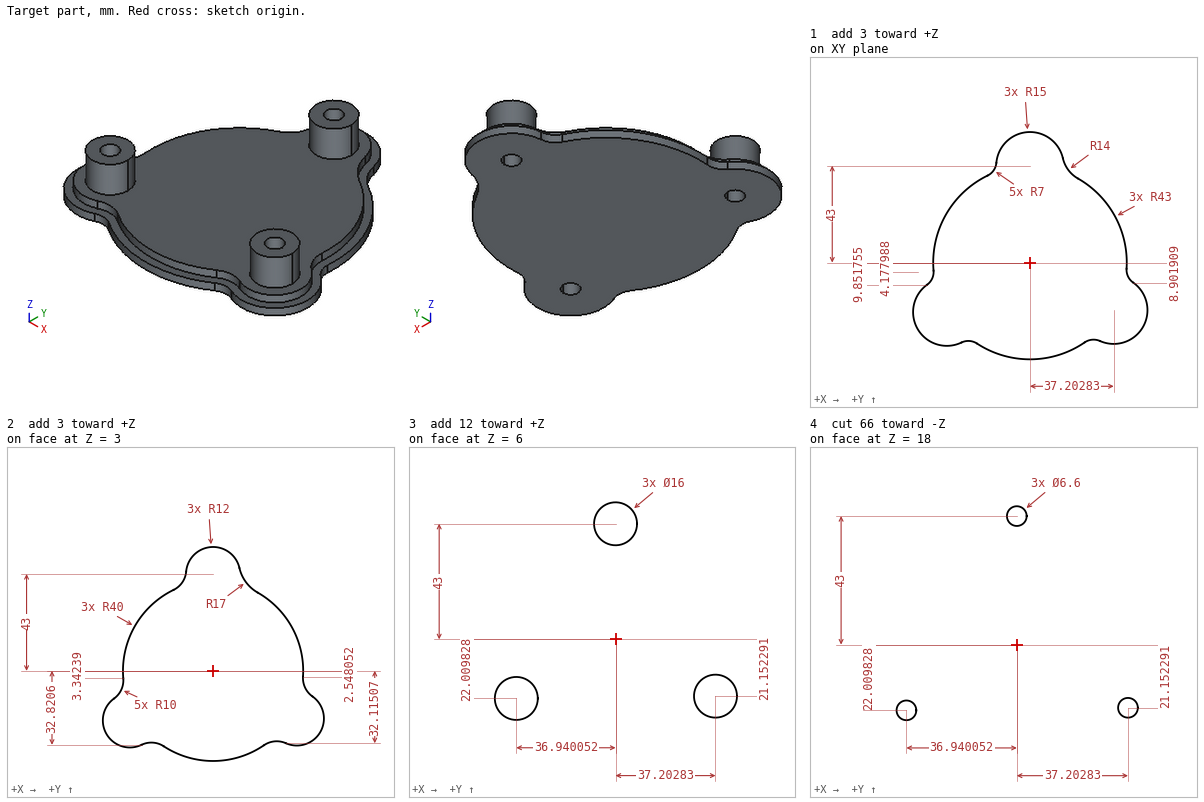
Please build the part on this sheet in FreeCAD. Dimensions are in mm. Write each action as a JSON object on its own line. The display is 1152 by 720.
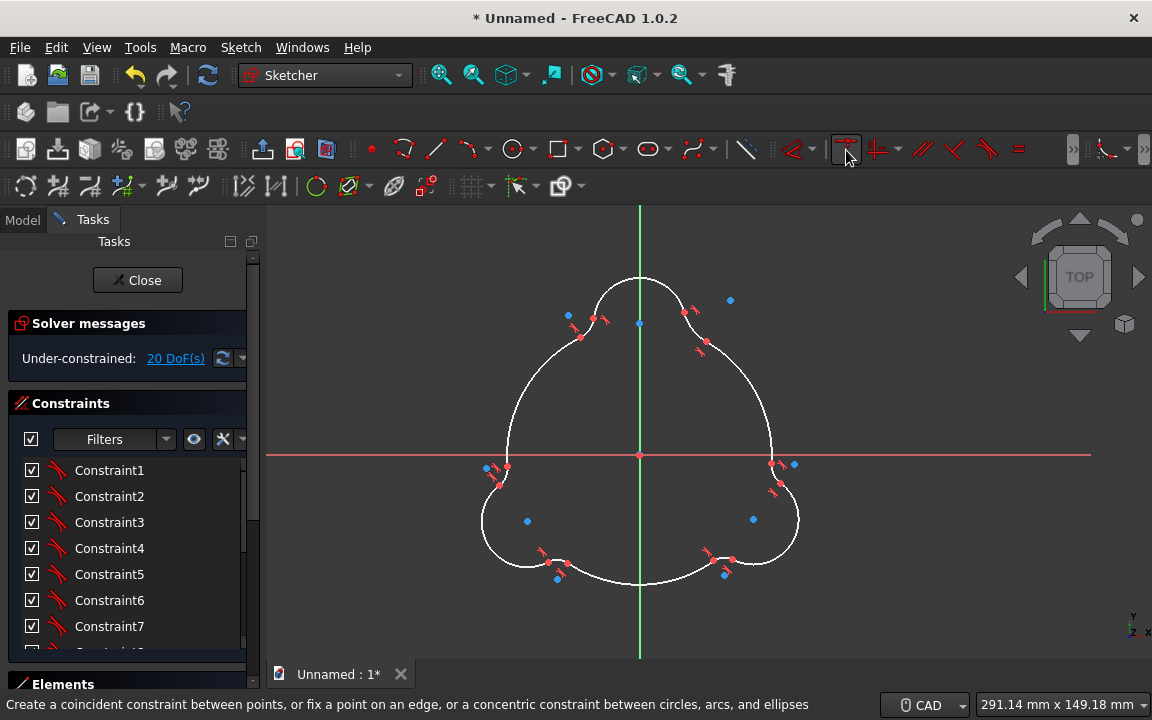
{"action": "scroll", "coordinate": [640, 455], "scroll_direction": "up", "scroll_amount": 4}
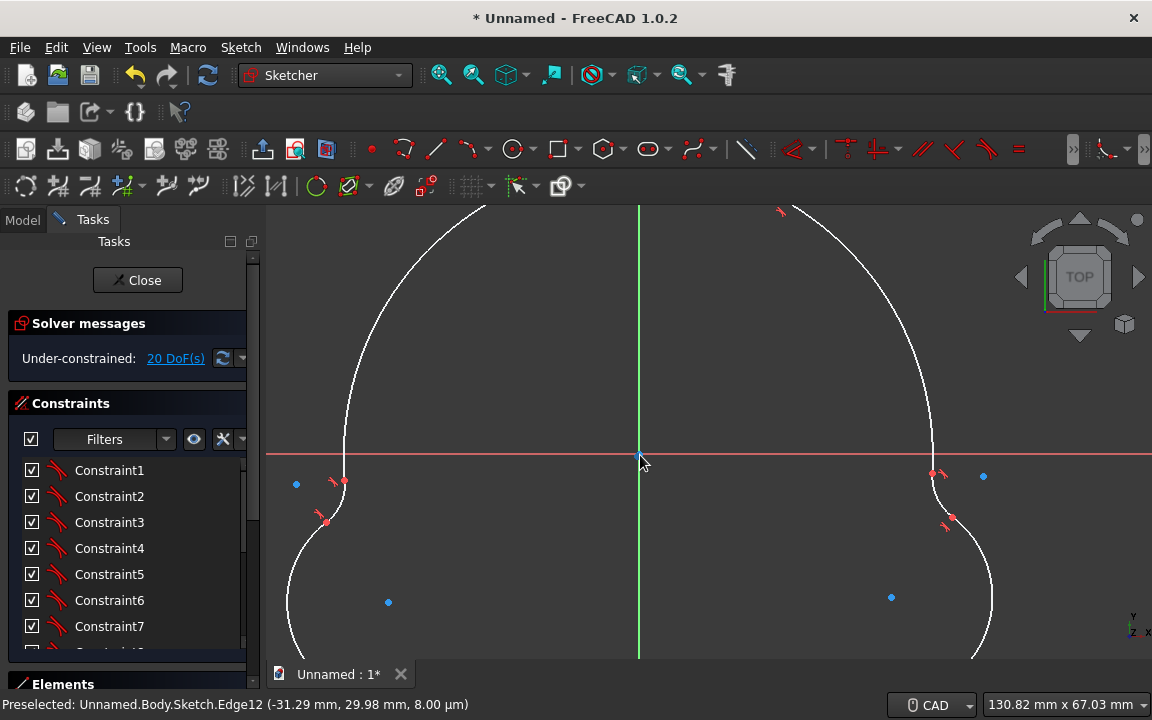
{"action": "left_click_drag", "start_coordinate": [628, 444], "coordinate": [649, 467]}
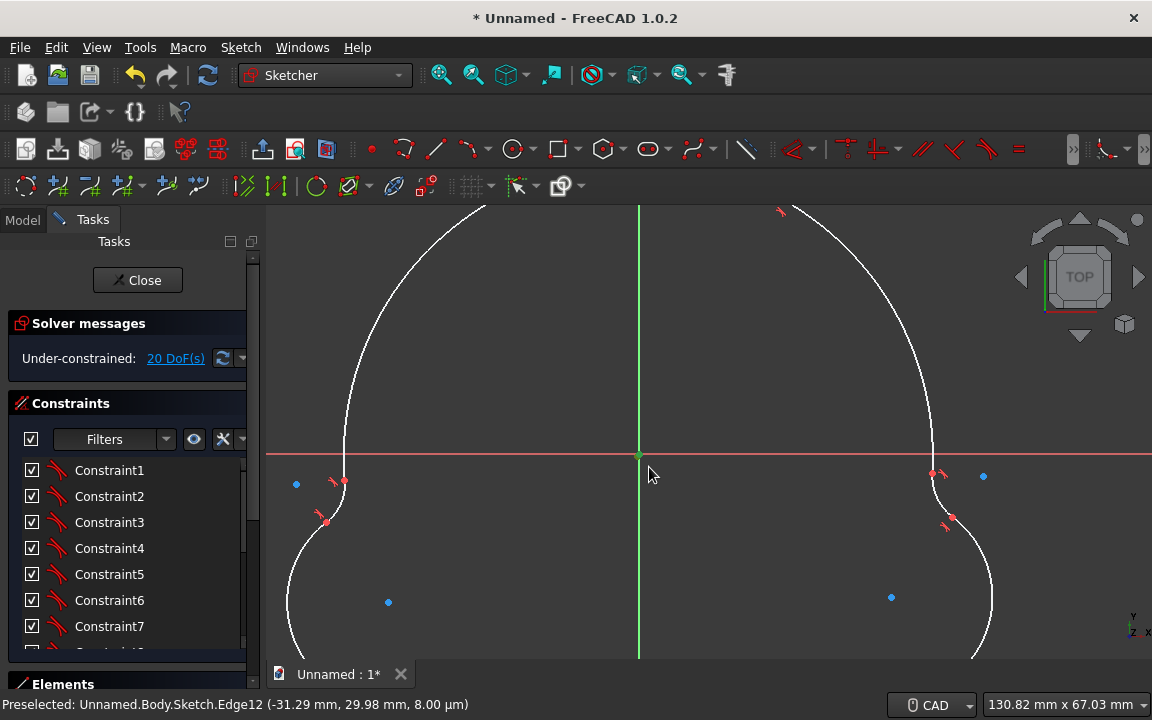
{"action": "key", "text": "c"}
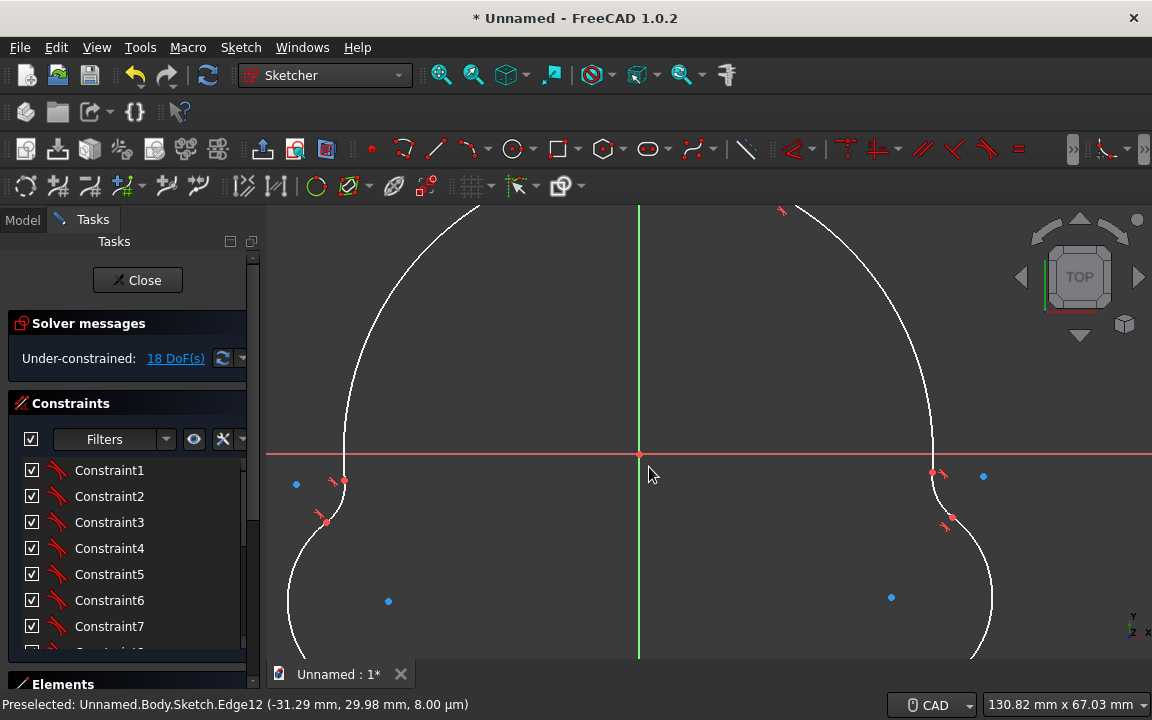
{"action": "left_click", "coordinate": [336, 512]}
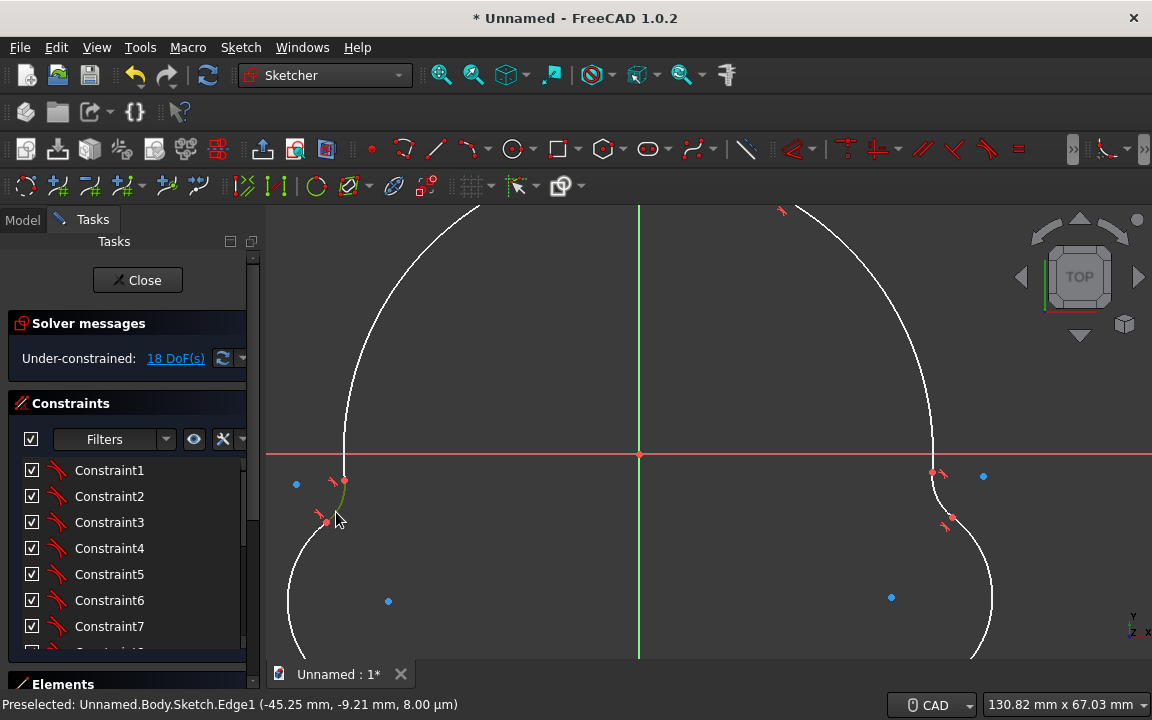
{"action": "scroll", "coordinate": [640, 455], "scroll_direction": "down", "scroll_amount": 4}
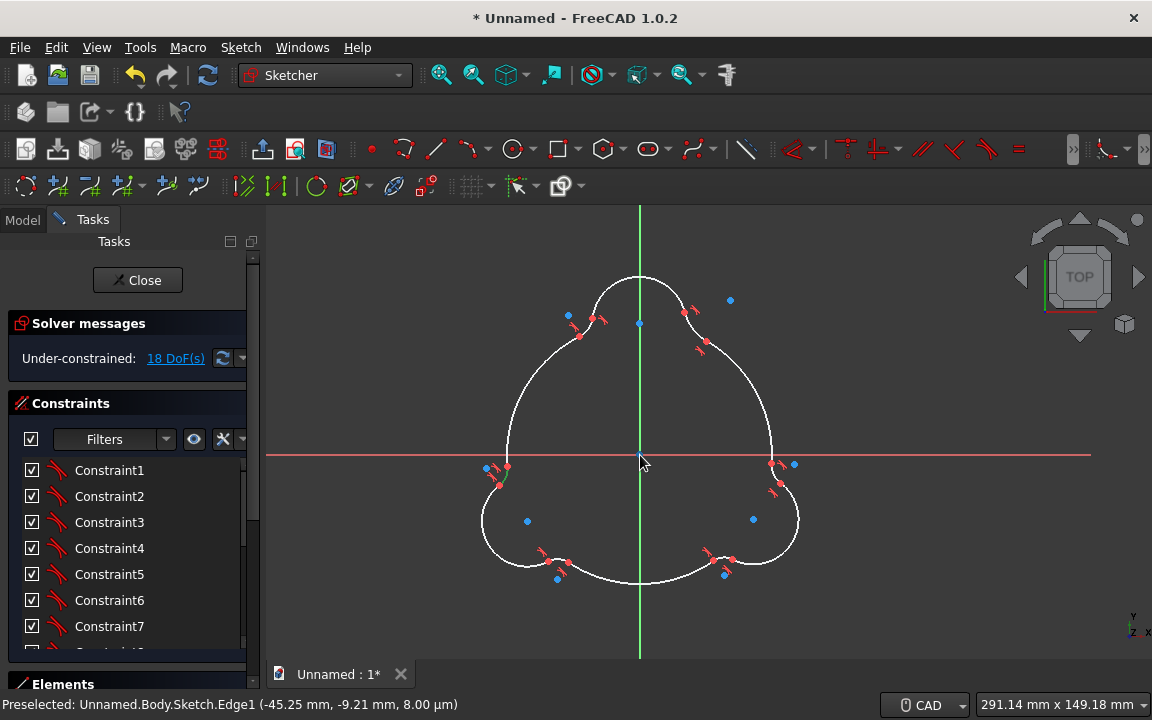
{"action": "scroll", "coordinate": [563, 560], "scroll_direction": "up", "scroll_amount": 4}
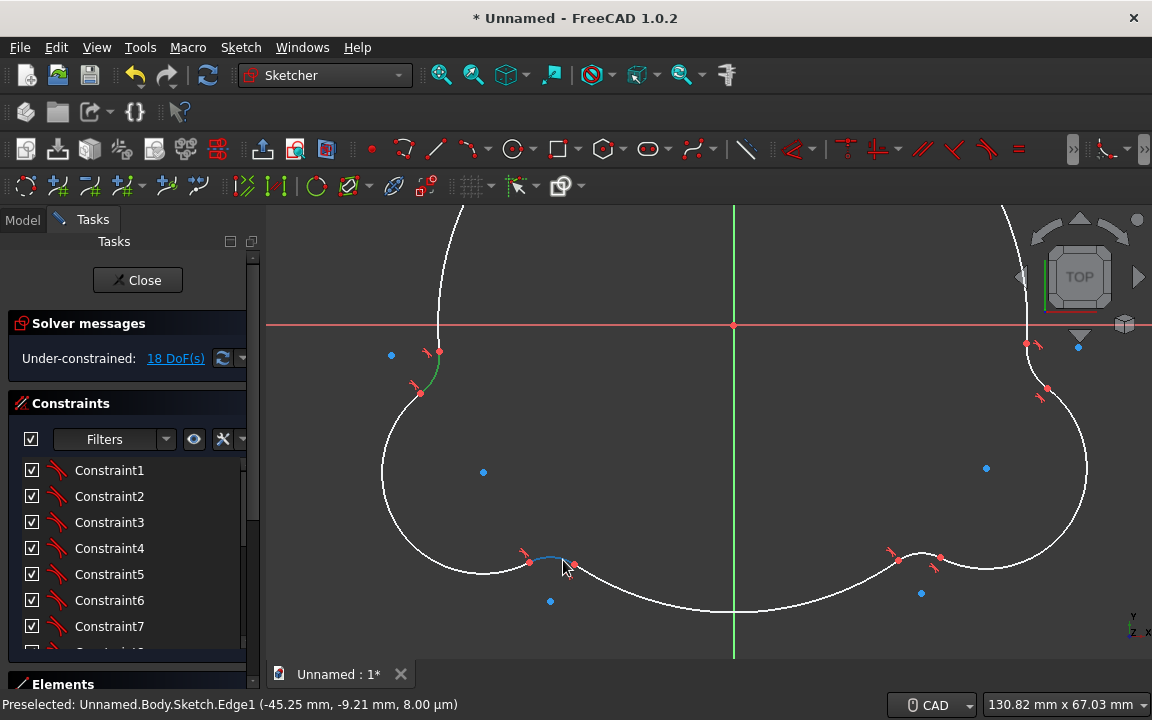
{"action": "left_click", "coordinate": [562, 559]}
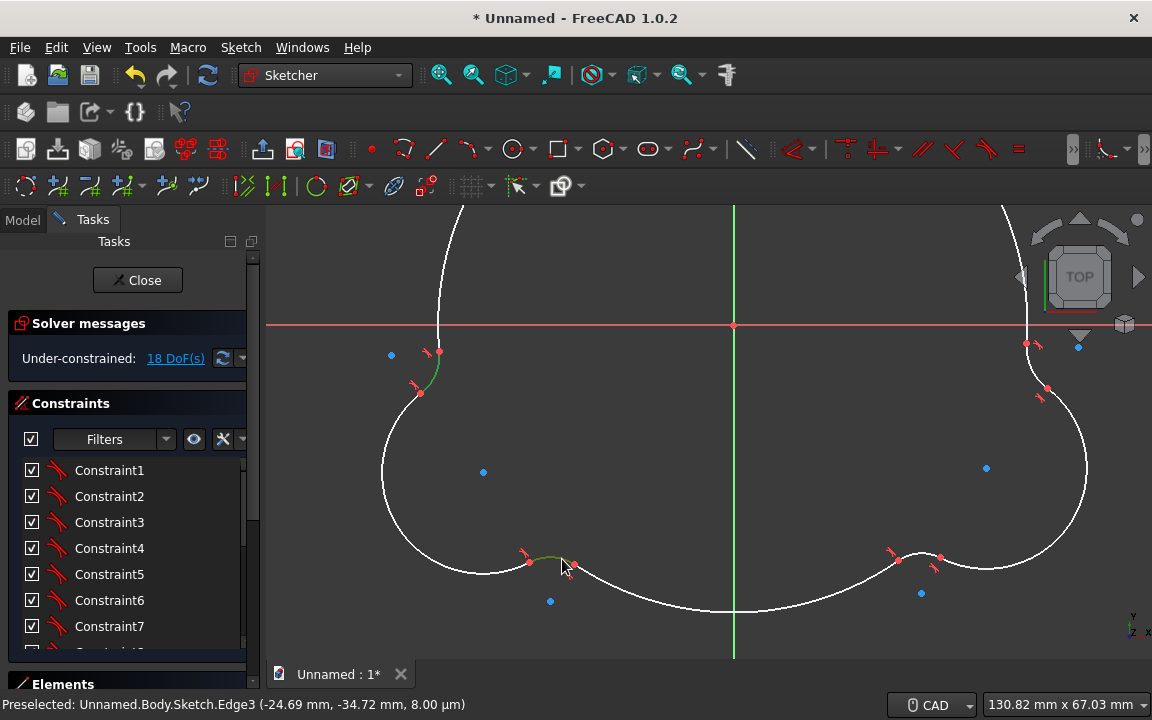
{"action": "left_click", "coordinate": [928, 554]}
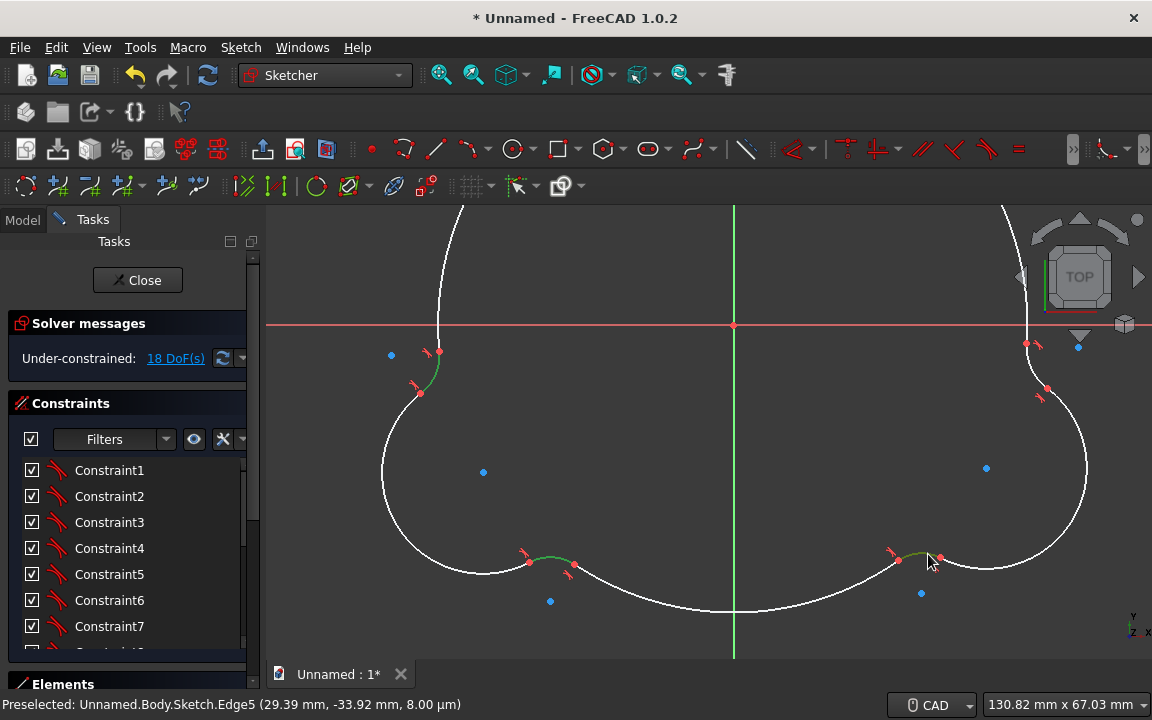
{"action": "scroll", "coordinate": [563, 561], "scroll_direction": "down", "scroll_amount": 4}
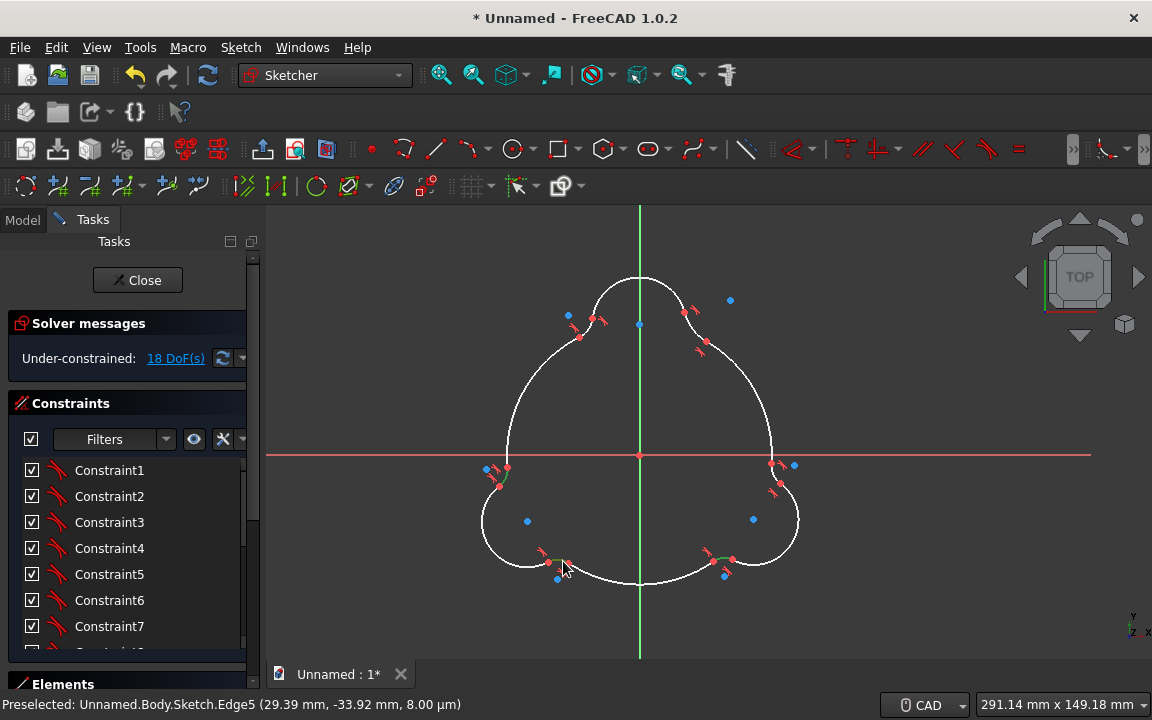
{"action": "scroll", "coordinate": [772, 471], "scroll_direction": "up", "scroll_amount": 4}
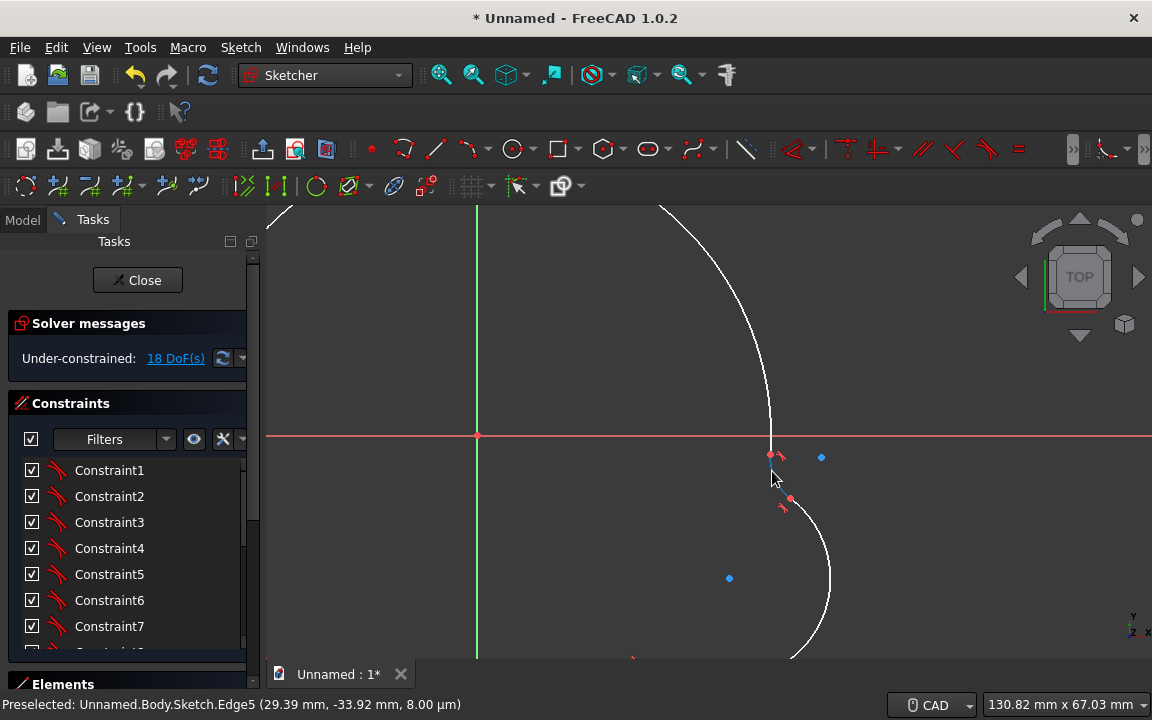
{"action": "left_click", "coordinate": [772, 469]}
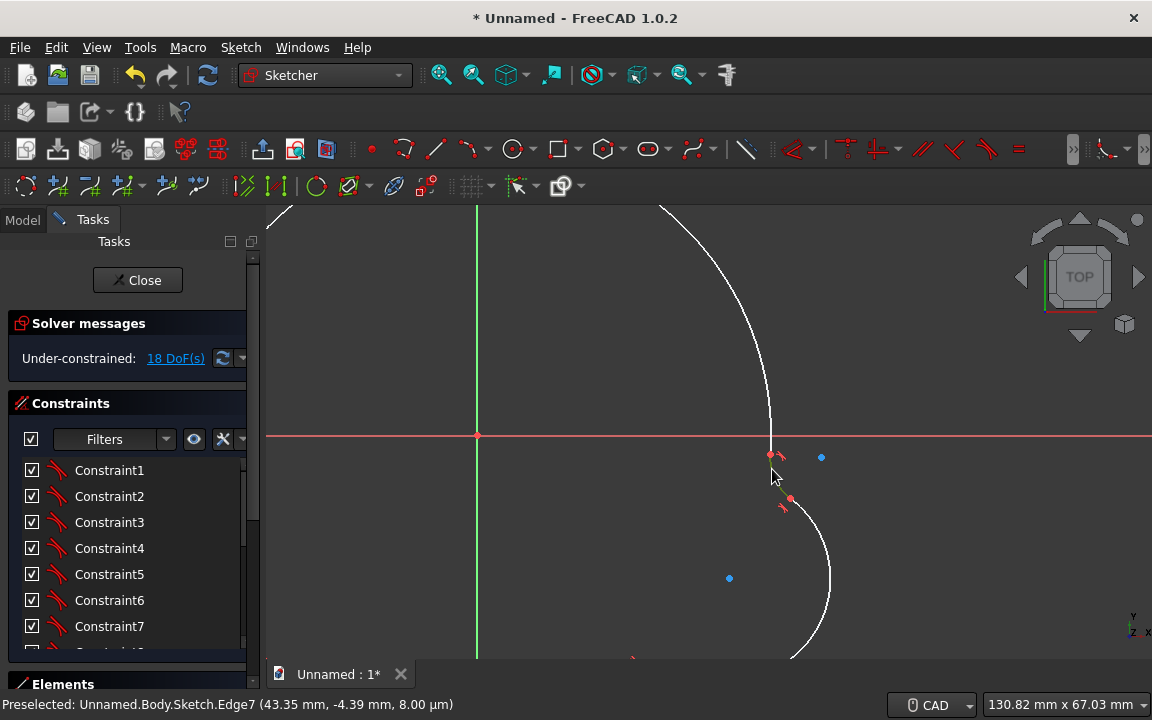
{"action": "scroll", "coordinate": [772, 470], "scroll_direction": "down", "scroll_amount": 4}